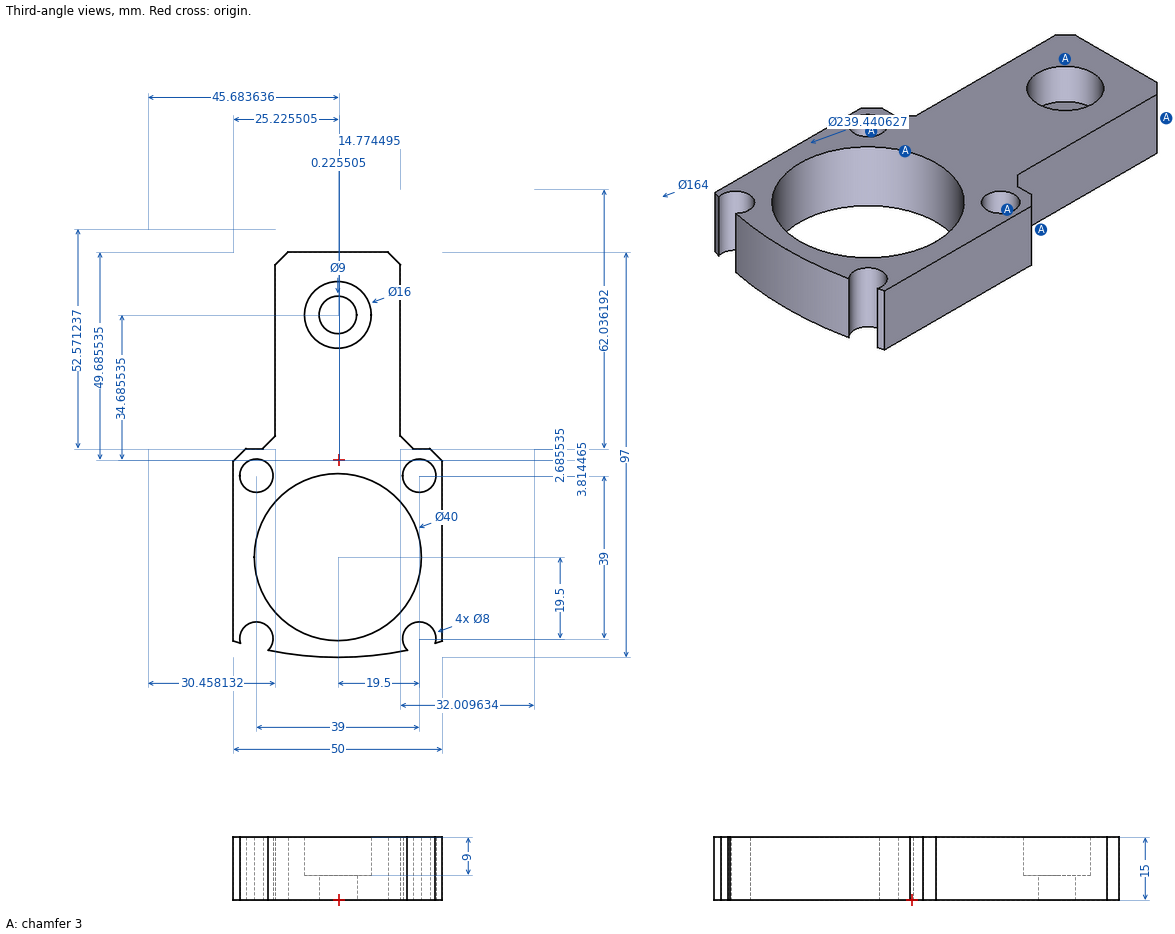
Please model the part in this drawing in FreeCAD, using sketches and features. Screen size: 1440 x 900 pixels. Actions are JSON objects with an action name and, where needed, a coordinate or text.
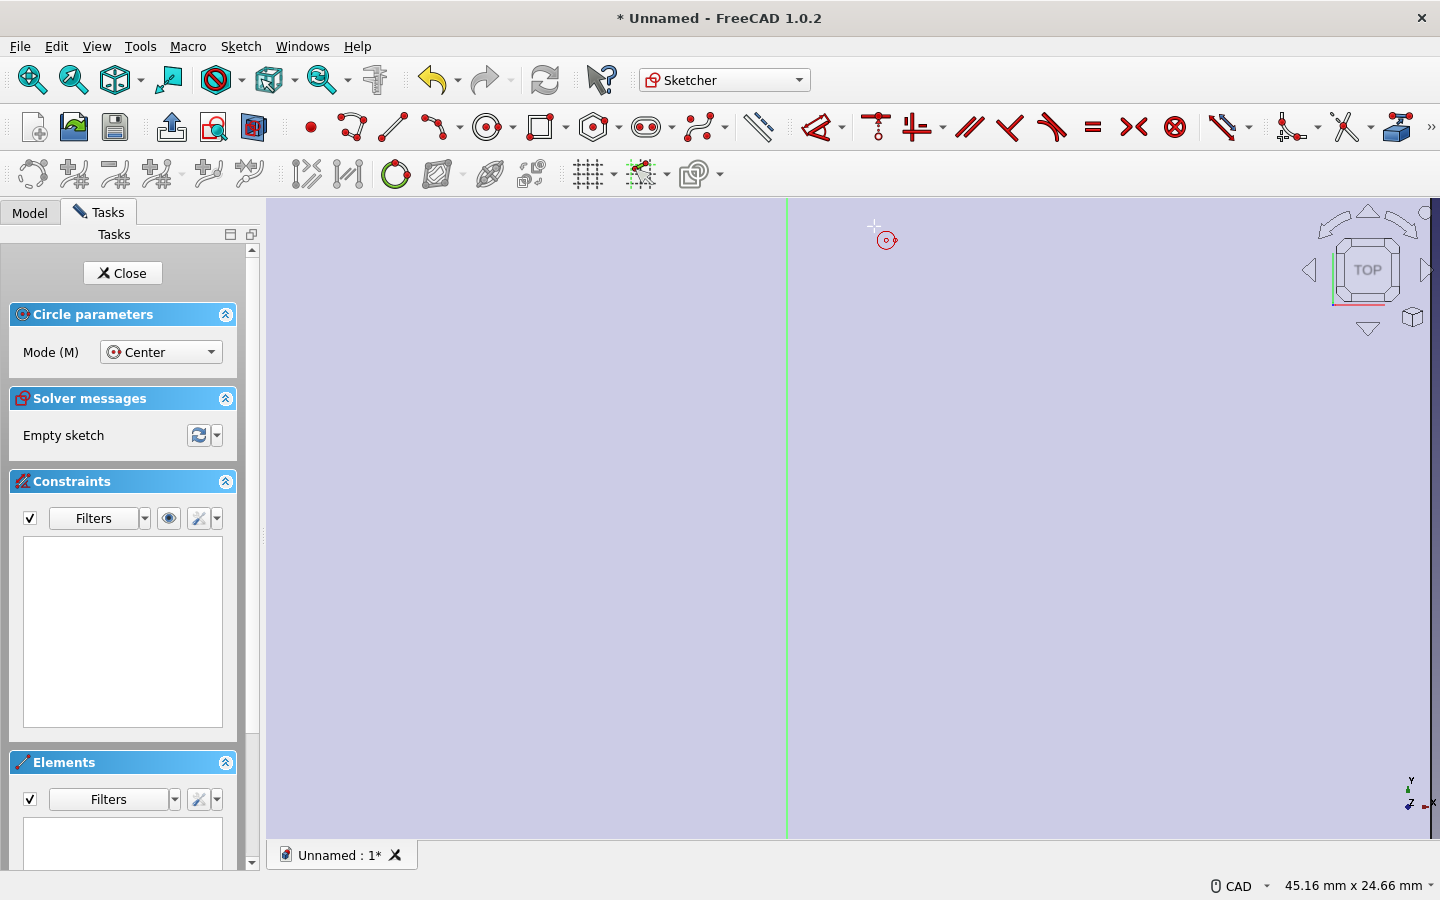
{"action": "scroll", "coordinate": [781, 510], "scroll_direction": "up", "scroll_amount": 5}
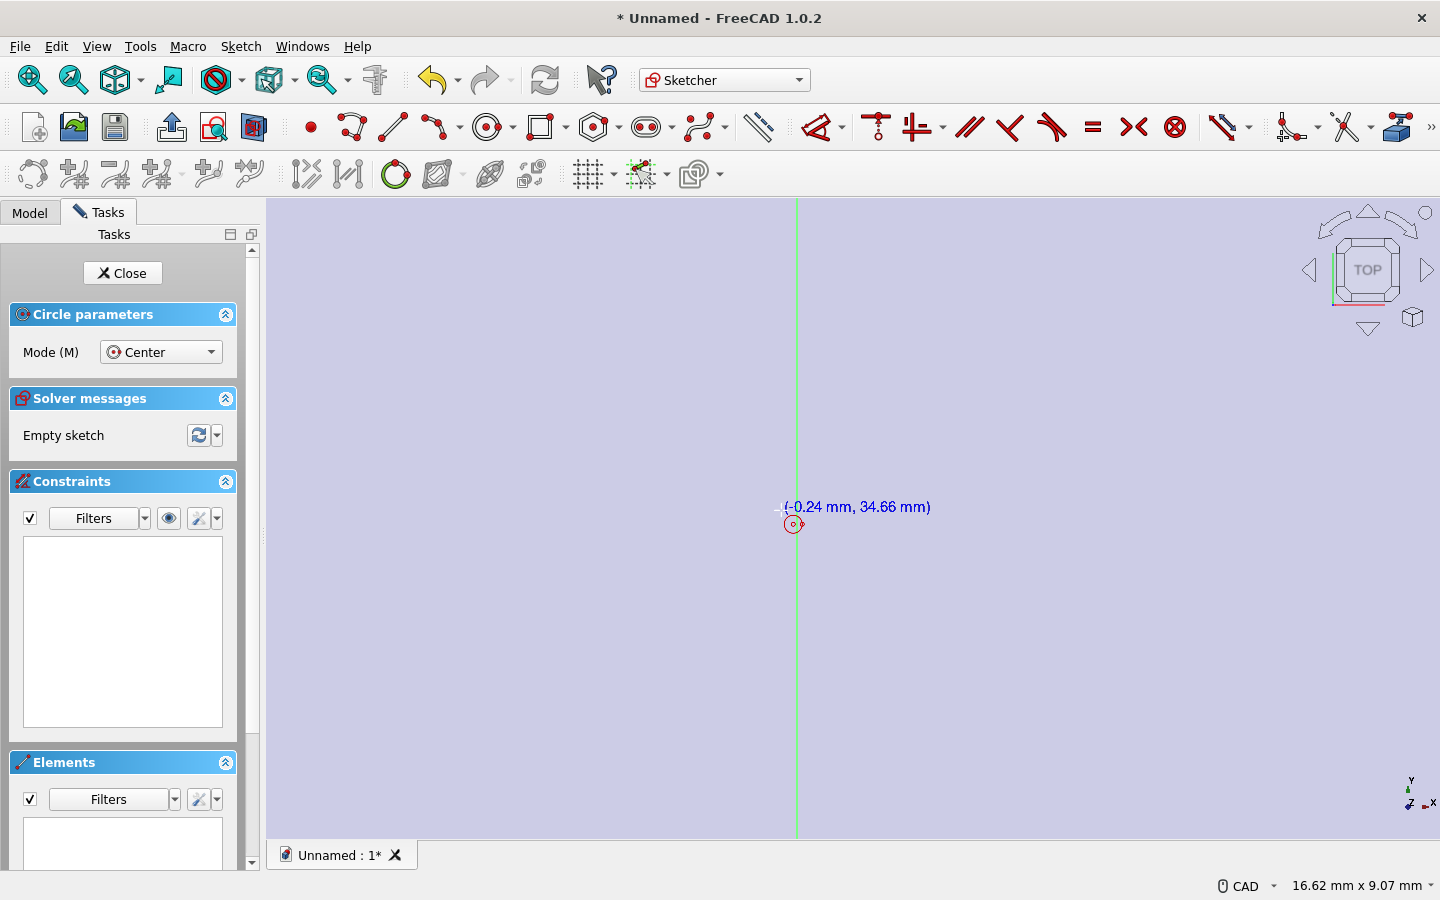
{"action": "left_click", "coordinate": [781, 510]}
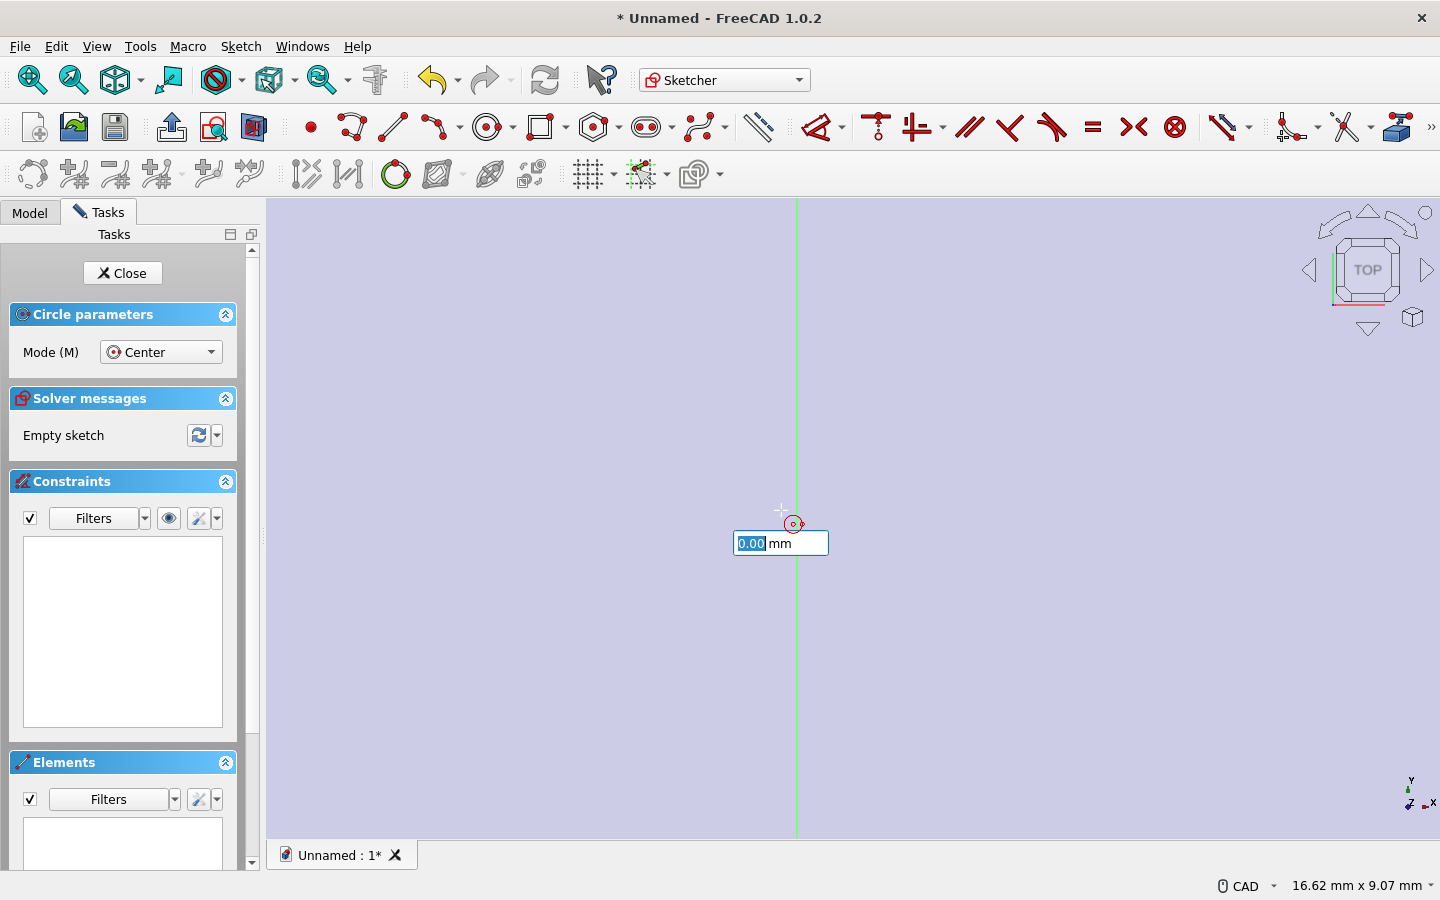
{"action": "scroll", "coordinate": [786, 523], "scroll_direction": "down", "scroll_amount": 5}
{"action": "mouse_move", "coordinate": [932, 372]}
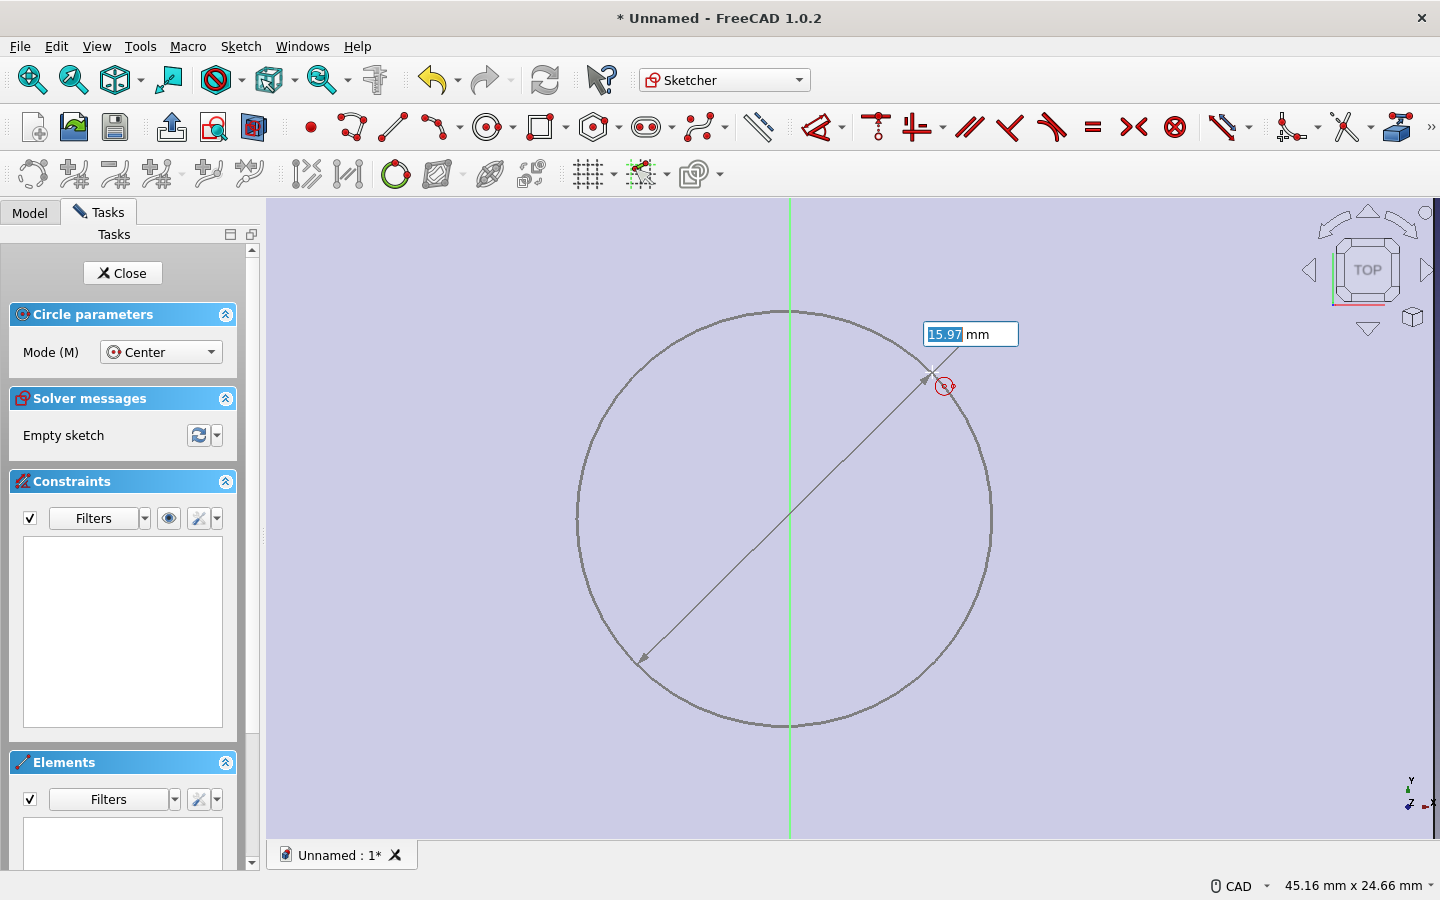
{"action": "type", "text": "16"}
{"action": "key", "text": "Return"}
{"action": "key", "text": "Escape"}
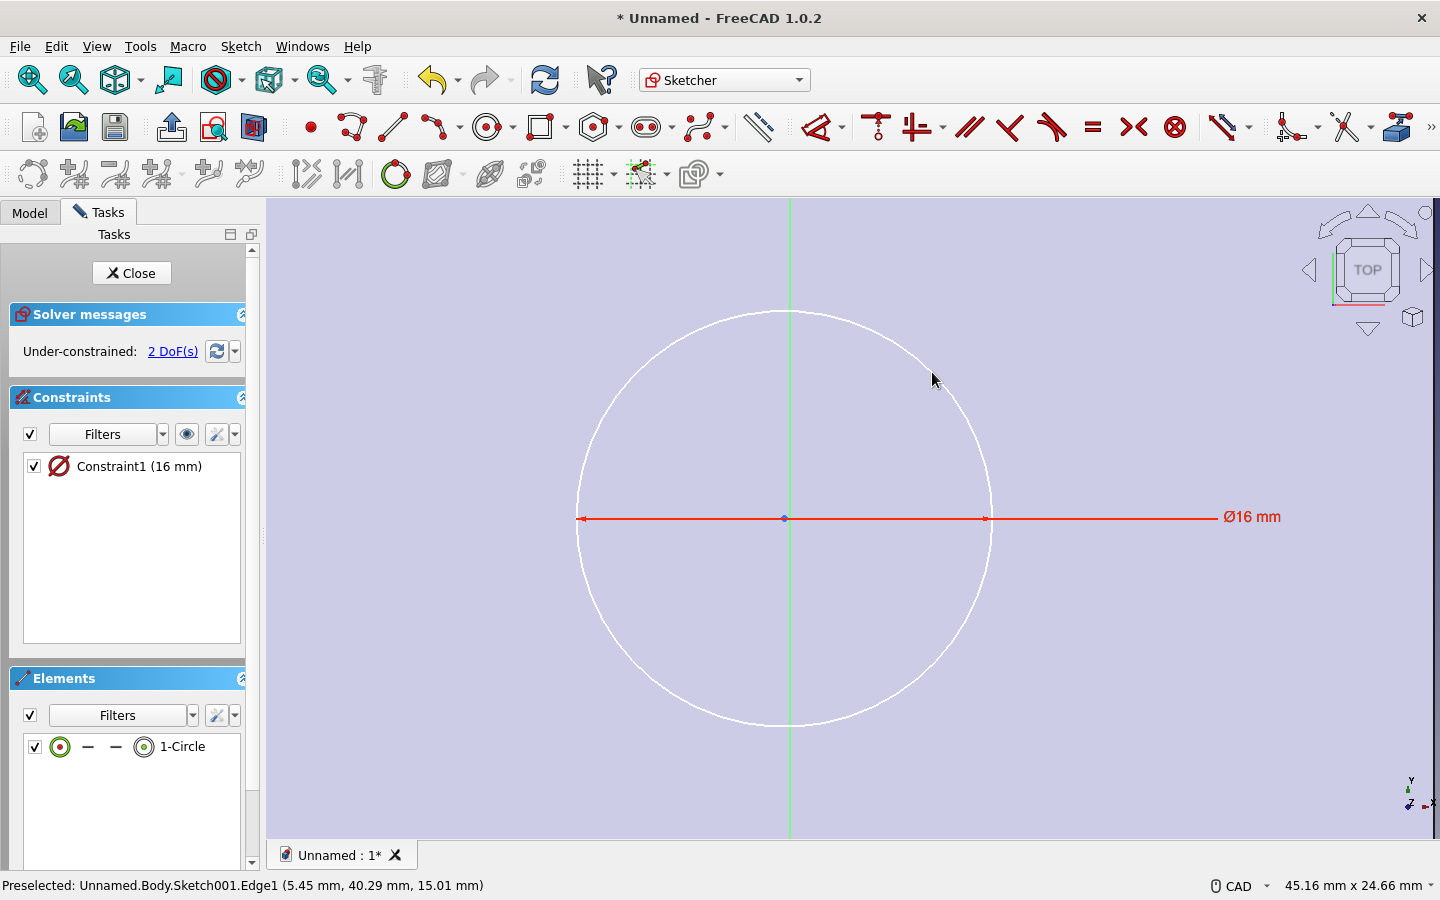
{"action": "key", "text": "d"}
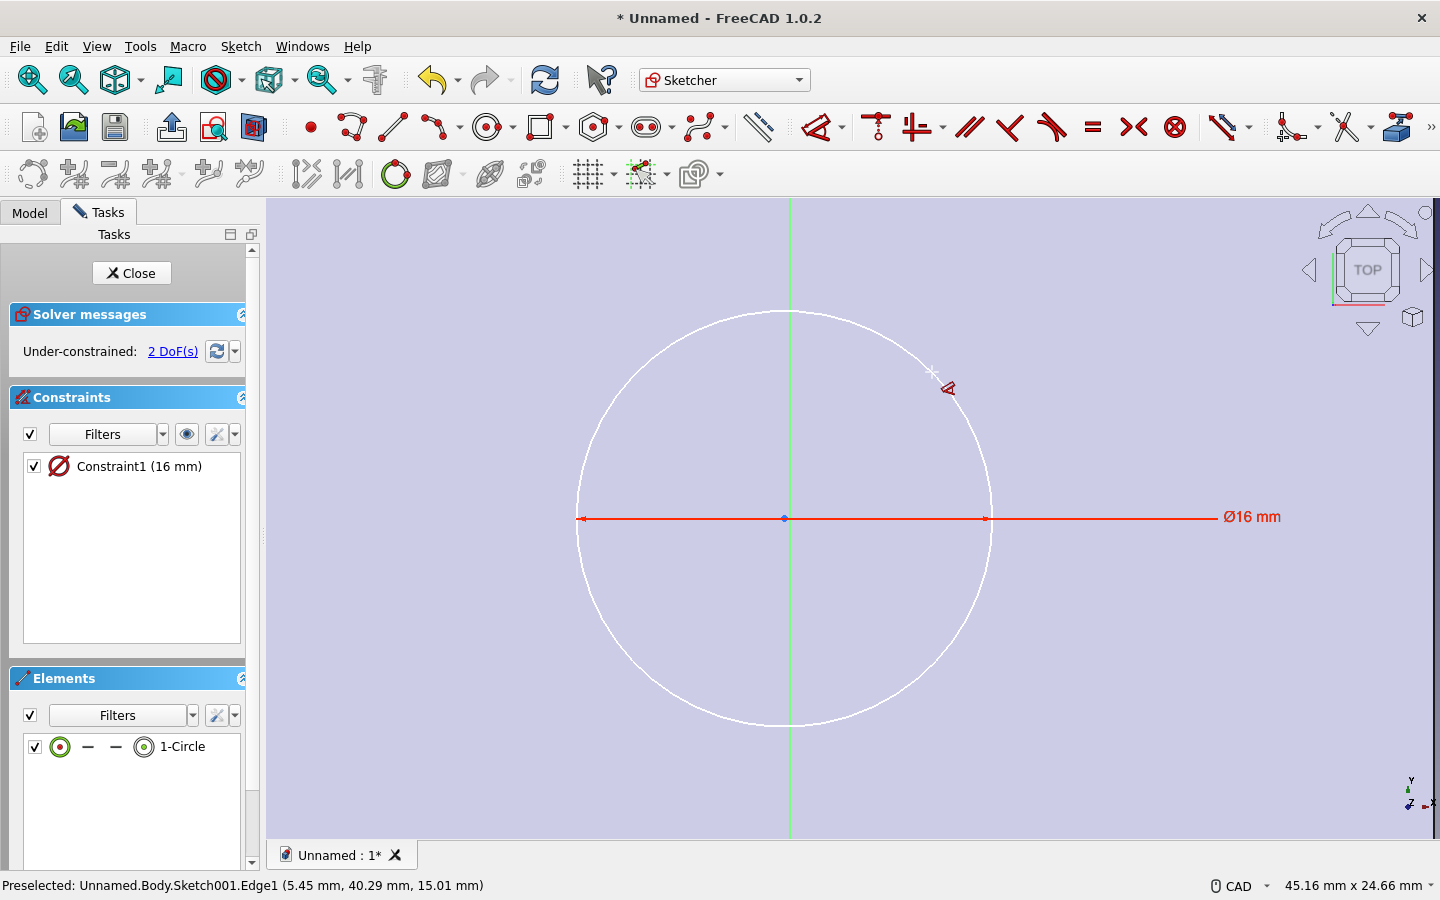
{"action": "scroll", "coordinate": [784, 519], "scroll_direction": "up", "scroll_amount": 10}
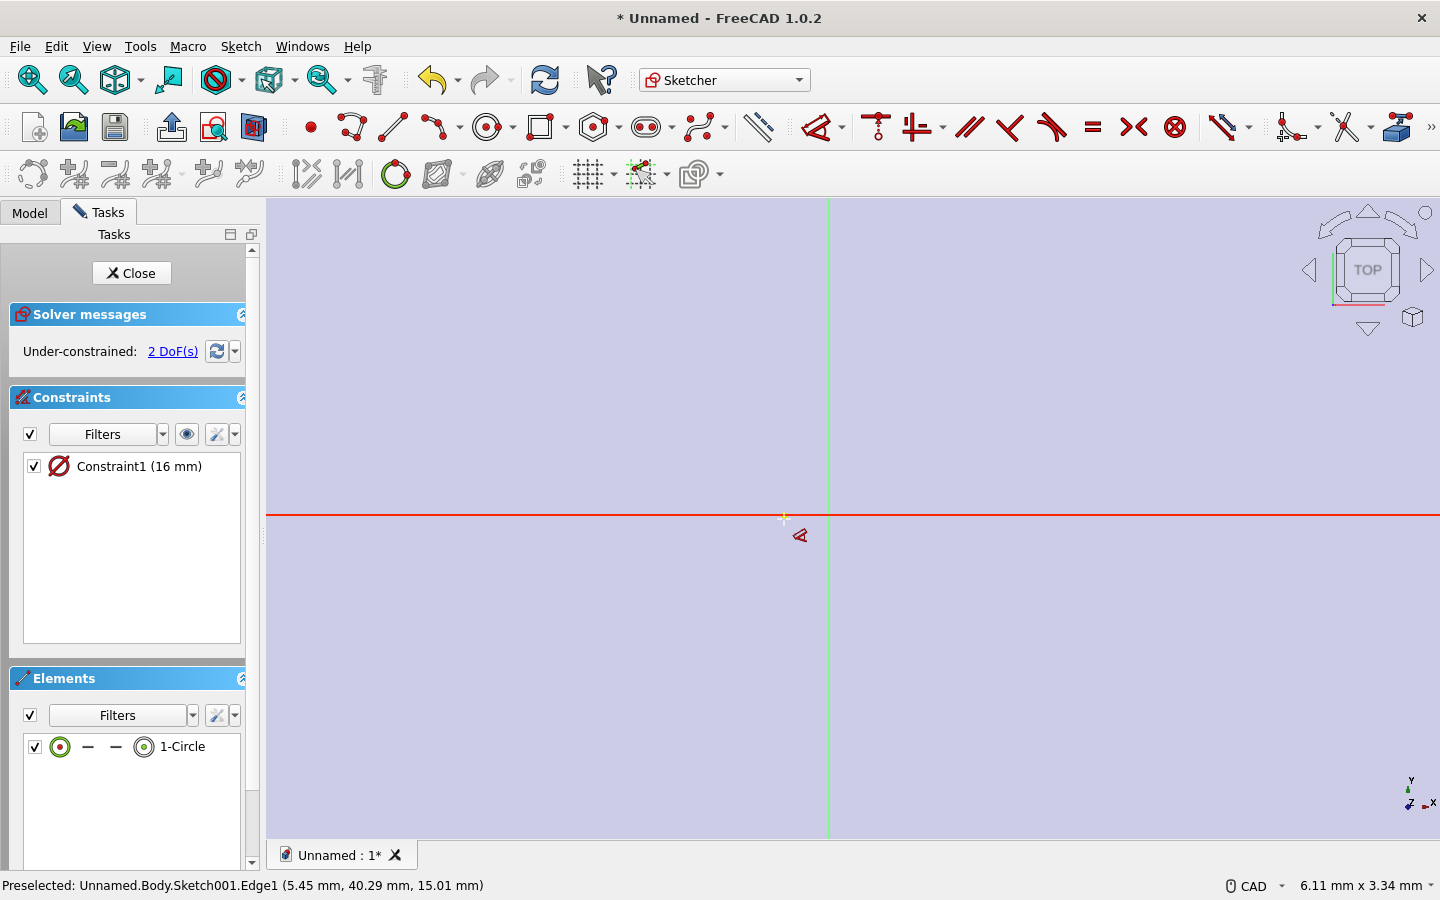
{"action": "left_click", "coordinate": [784, 515]}
{"action": "left_click", "coordinate": [807, 481]}